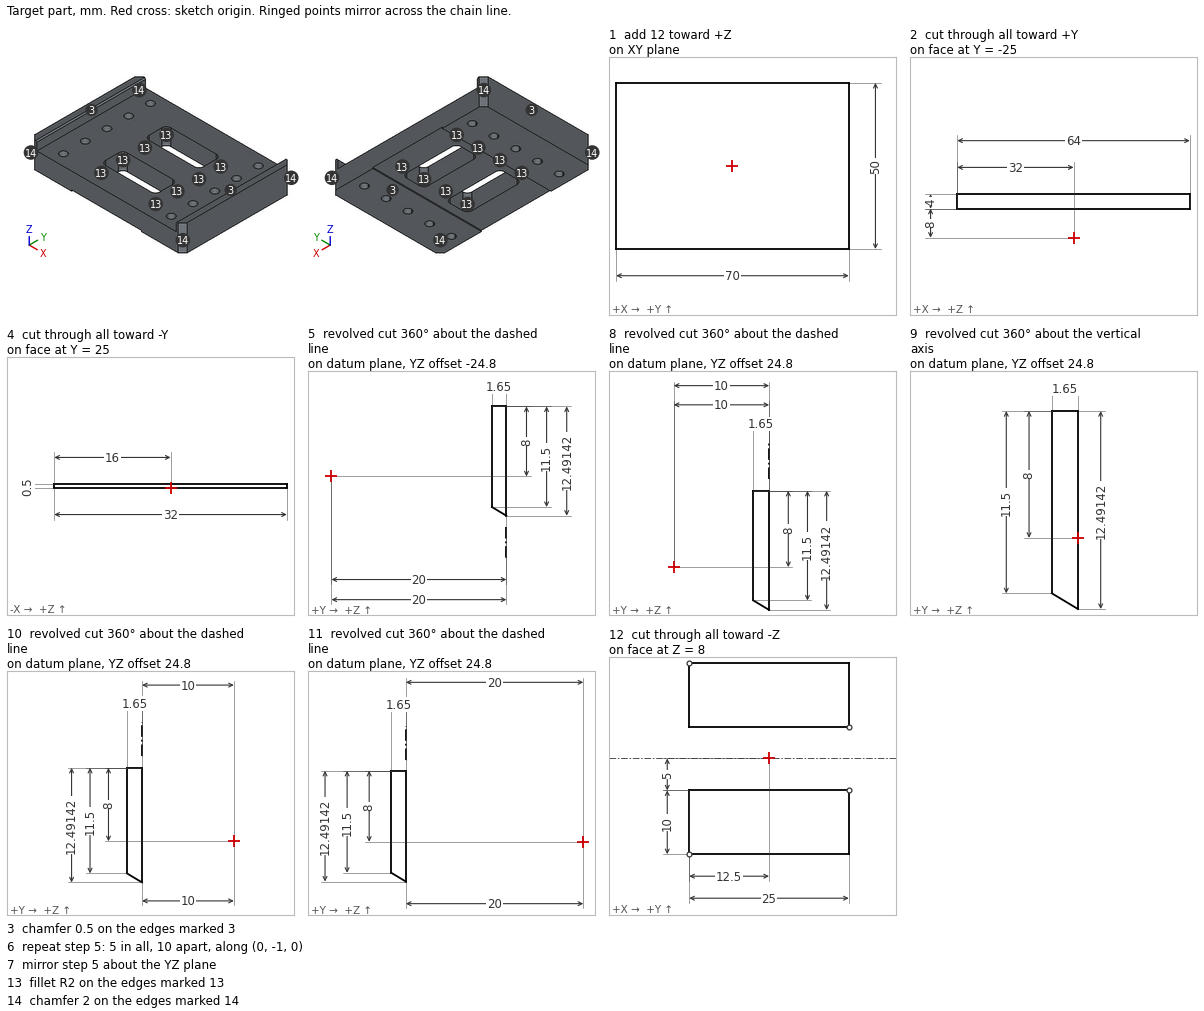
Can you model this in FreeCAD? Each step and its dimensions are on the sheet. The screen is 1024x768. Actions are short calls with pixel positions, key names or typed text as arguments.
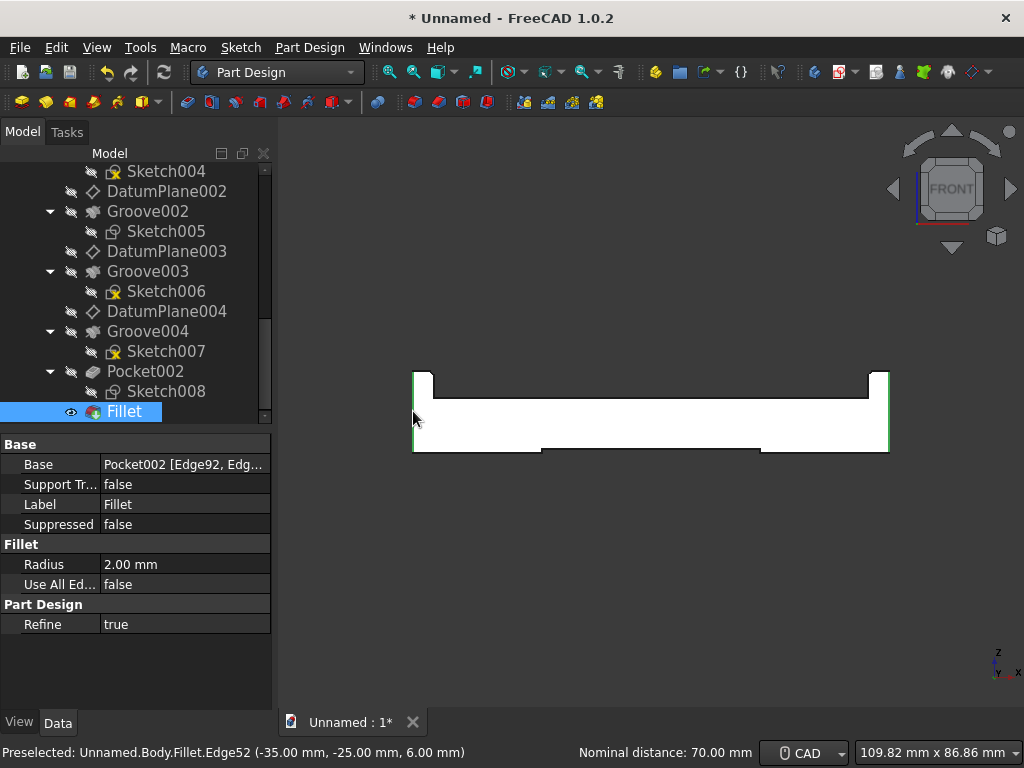
key(3)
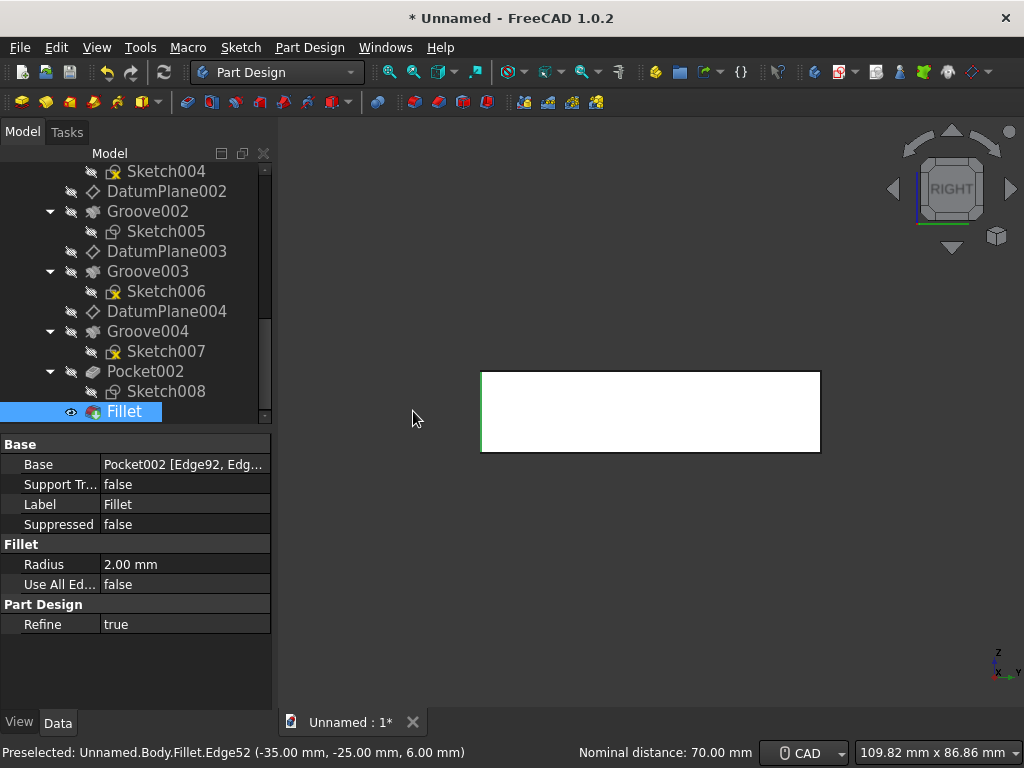
click(821, 411, ctrl)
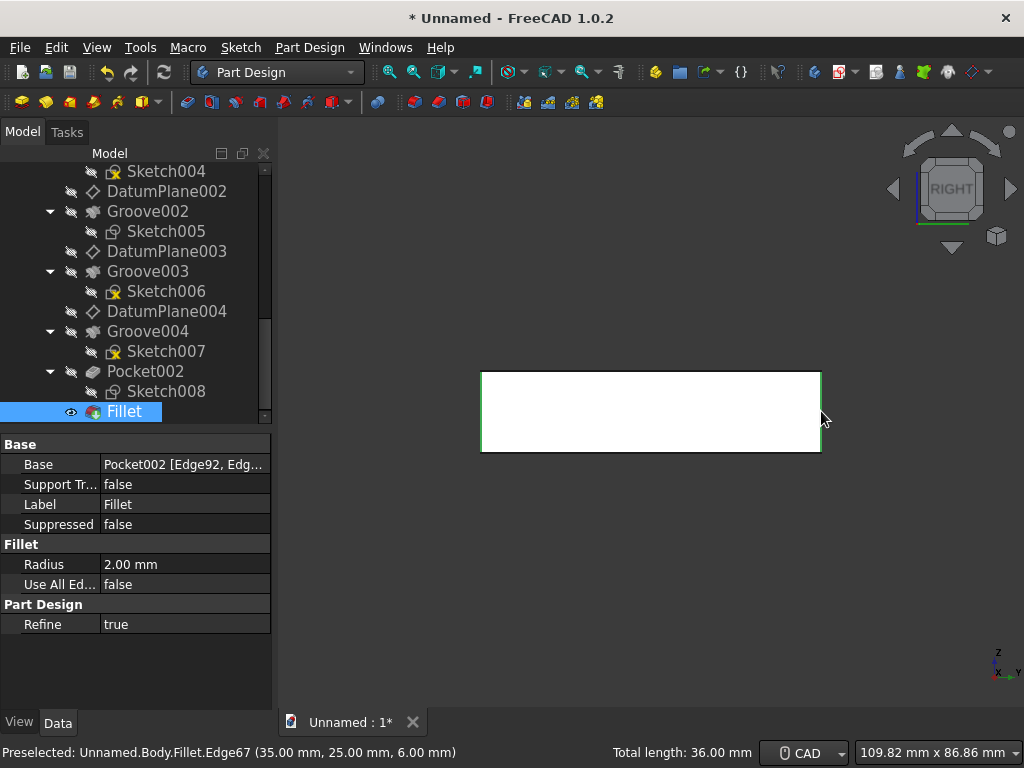
key(5)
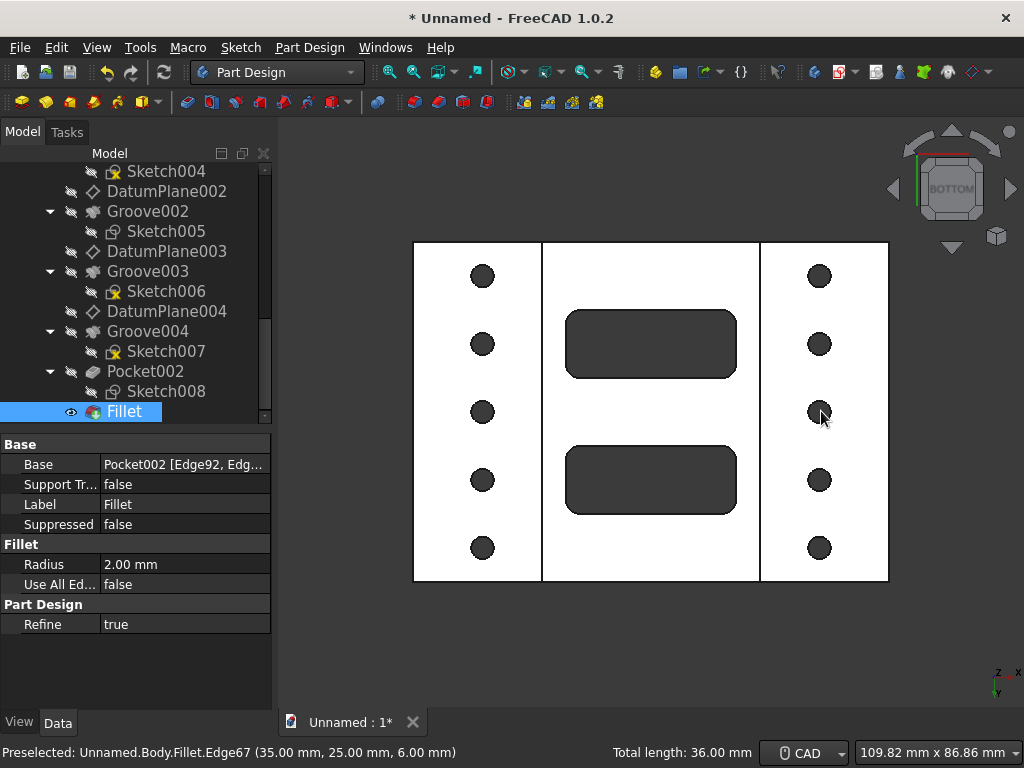
key(4)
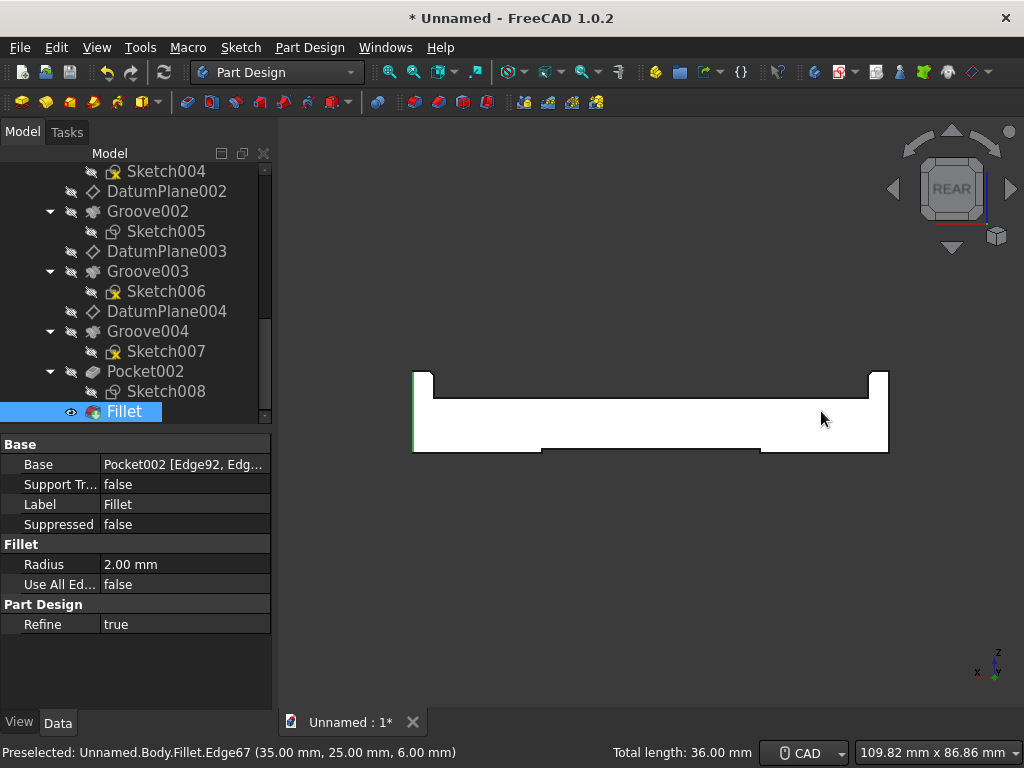
click(889, 411, ctrl)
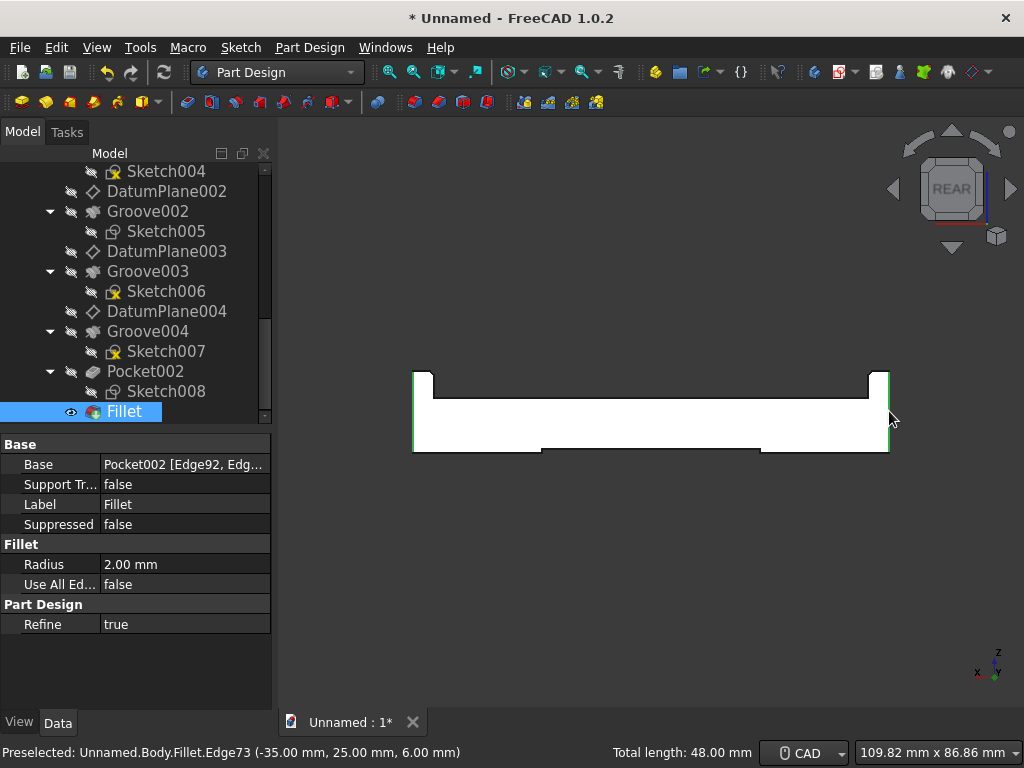
click(440, 102)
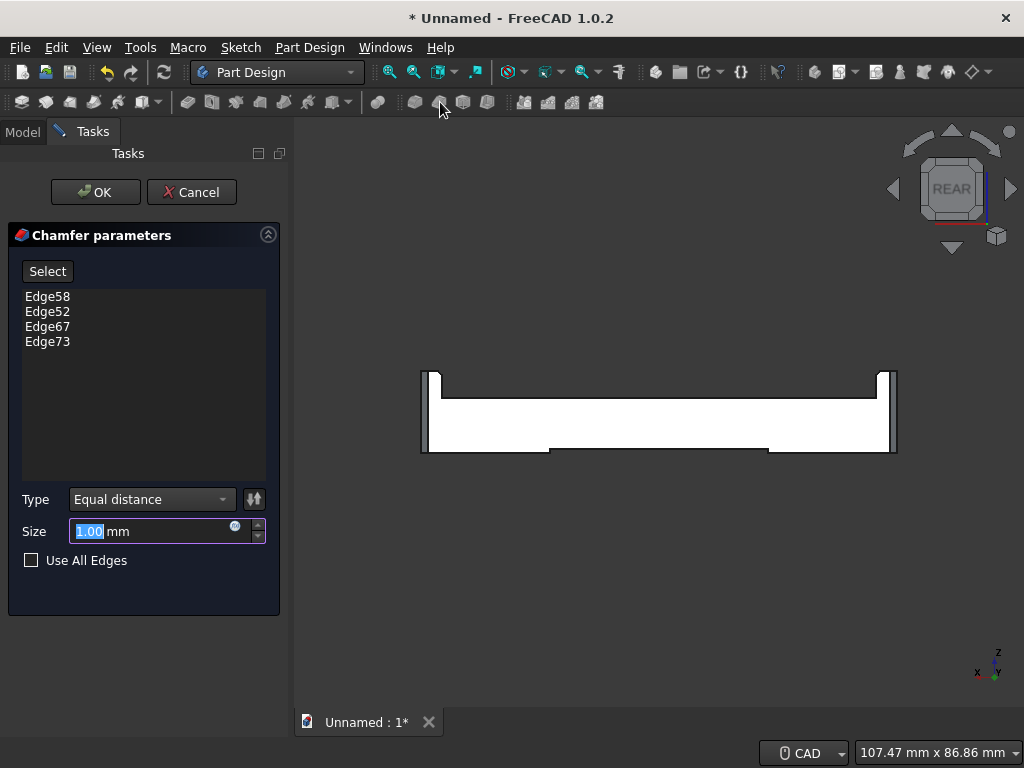
text(2)
key(Tab)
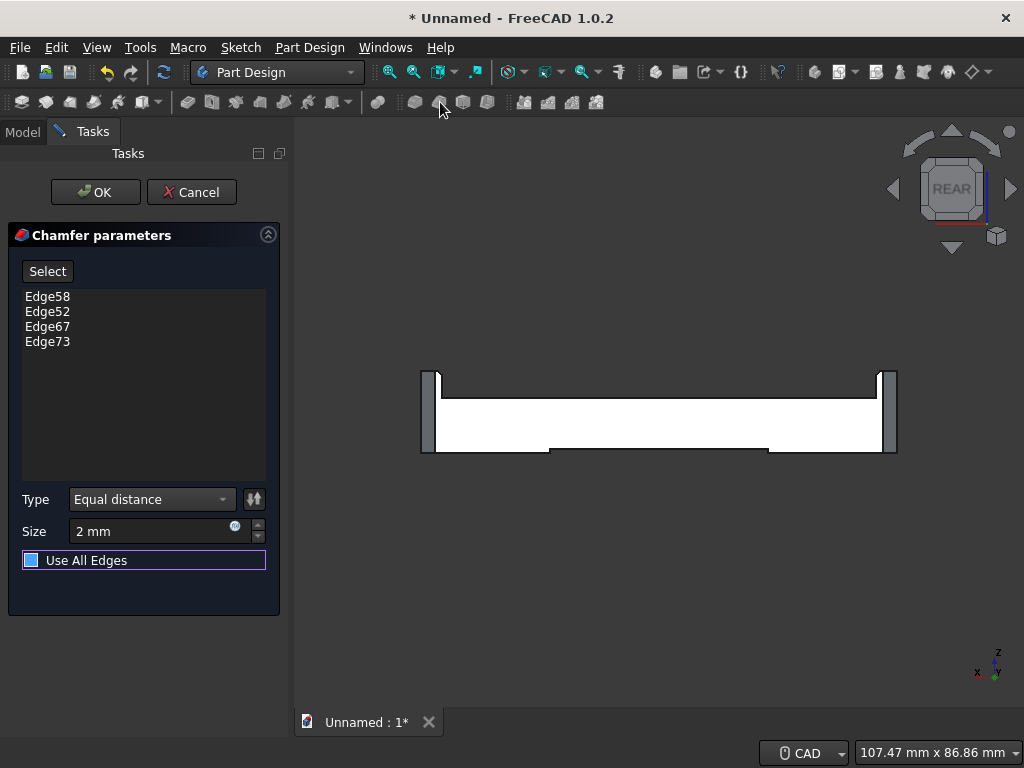
click(96, 192)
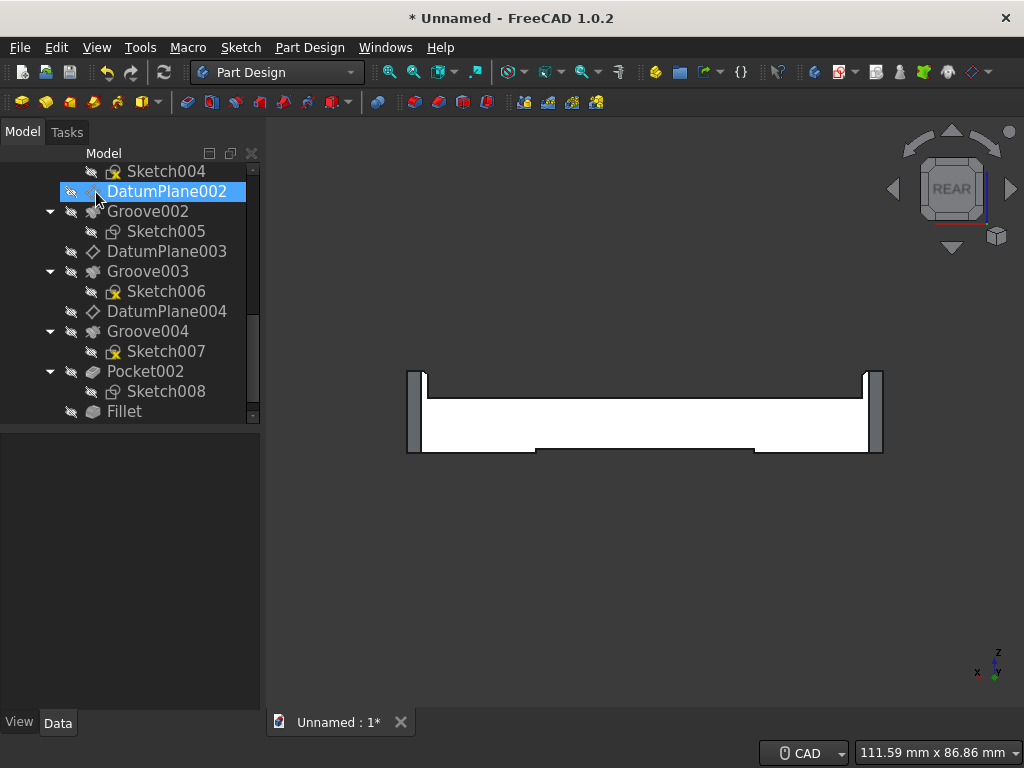
key(0)